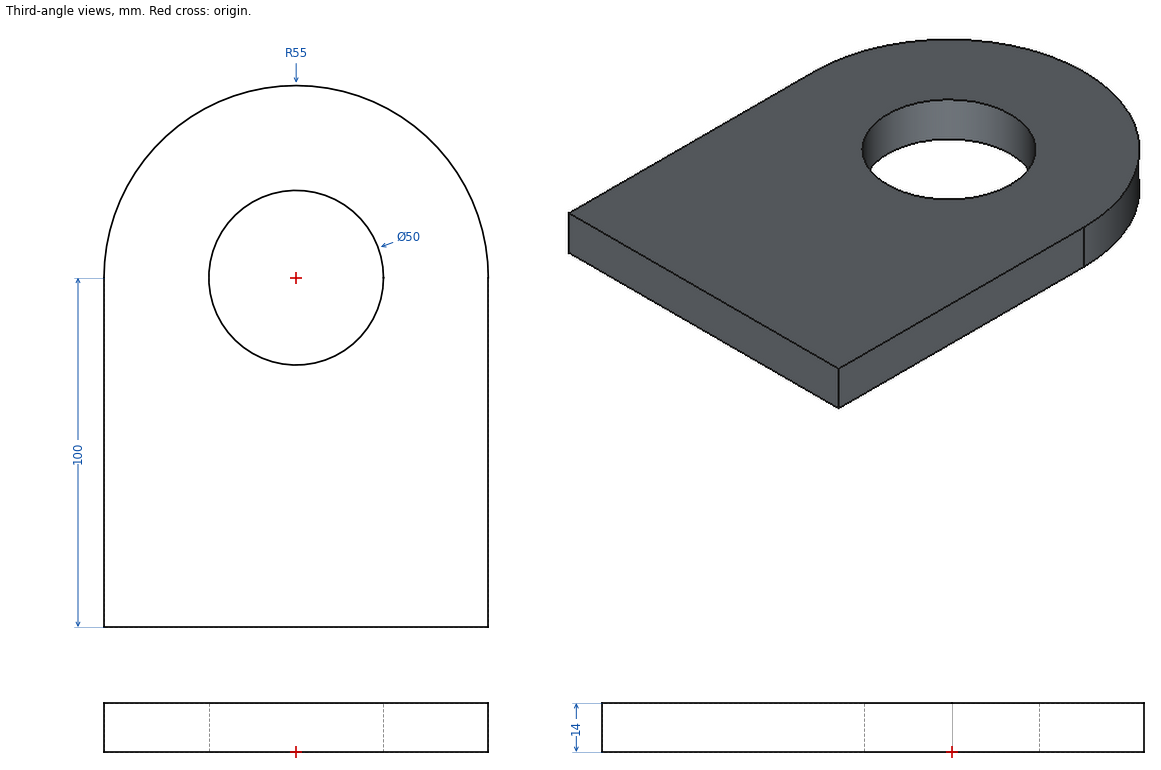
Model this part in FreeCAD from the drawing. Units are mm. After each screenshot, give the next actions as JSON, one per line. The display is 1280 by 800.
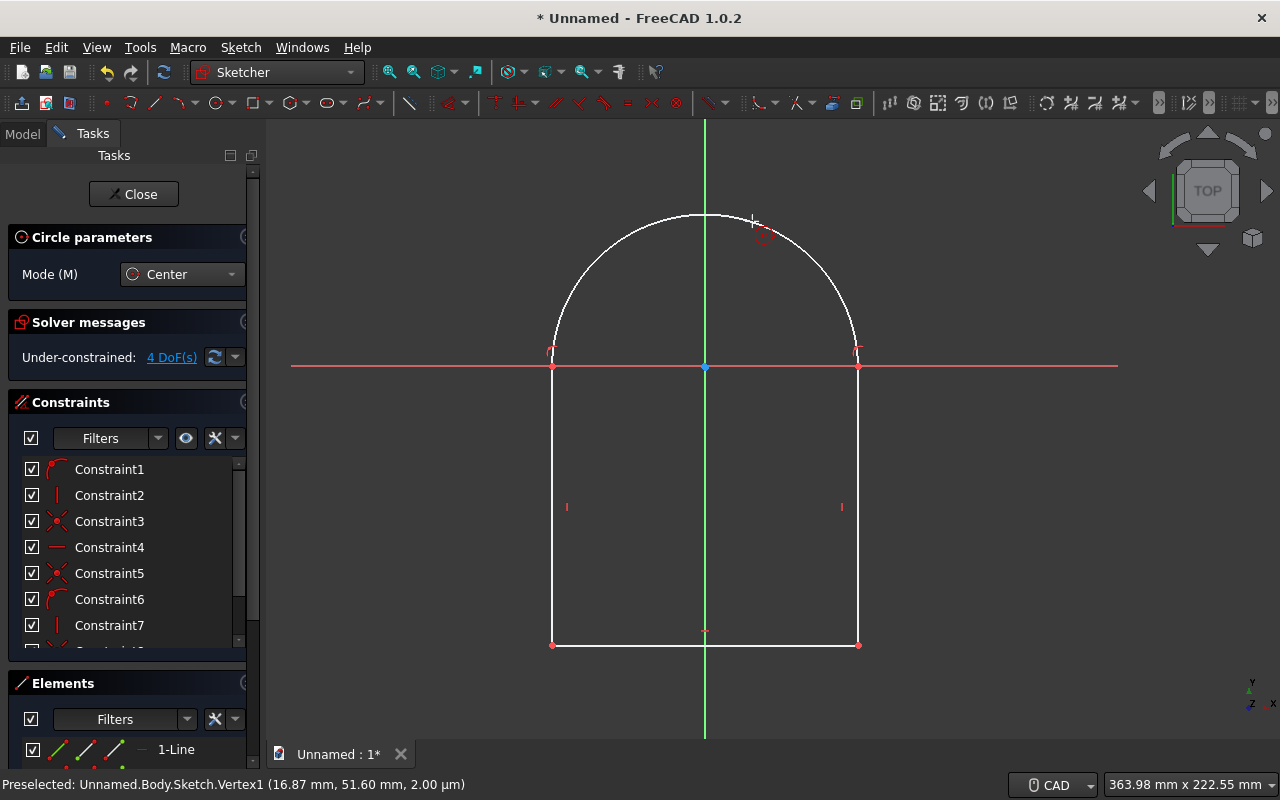
{"action": "left_click", "coordinate": [705, 366]}
{"action": "mouse_move", "coordinate": [754, 317]}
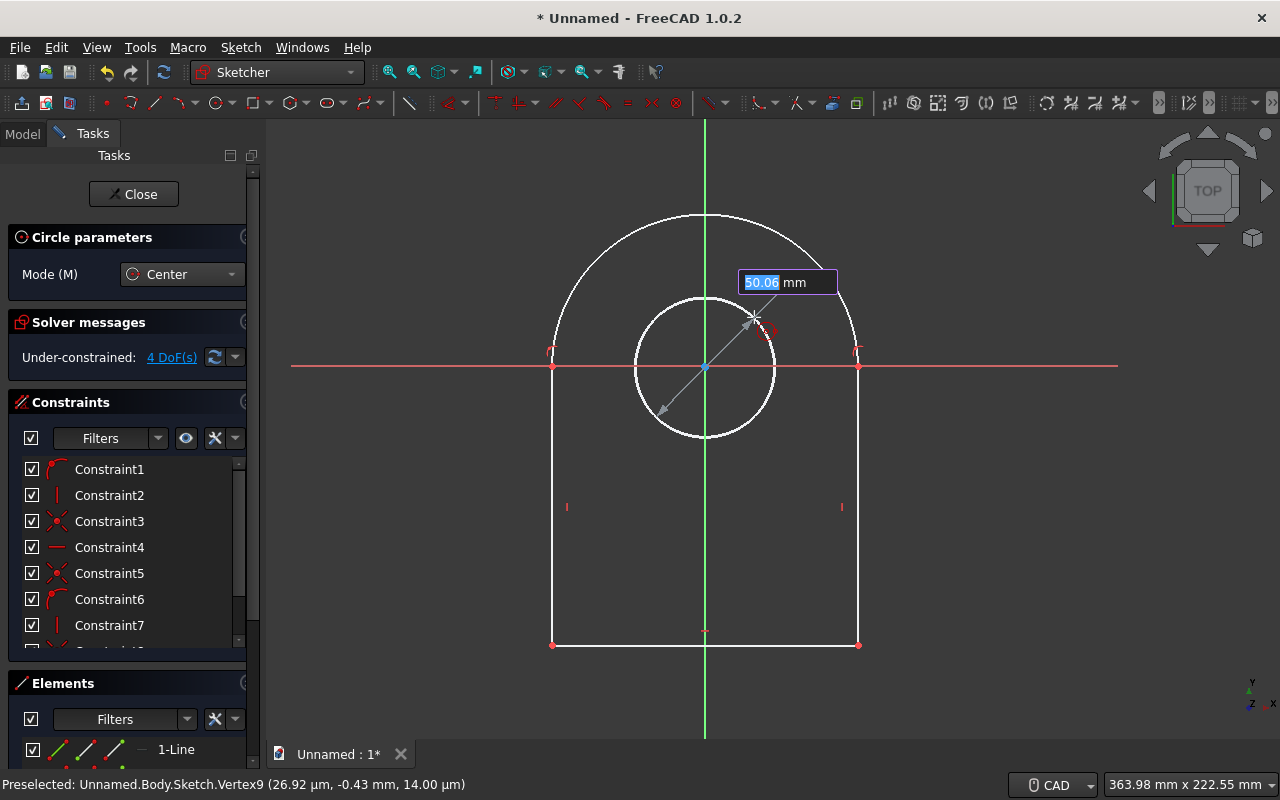
{"action": "type", "text": "50"}
{"action": "key", "text": "Return"}
{"action": "key", "text": "Escape"}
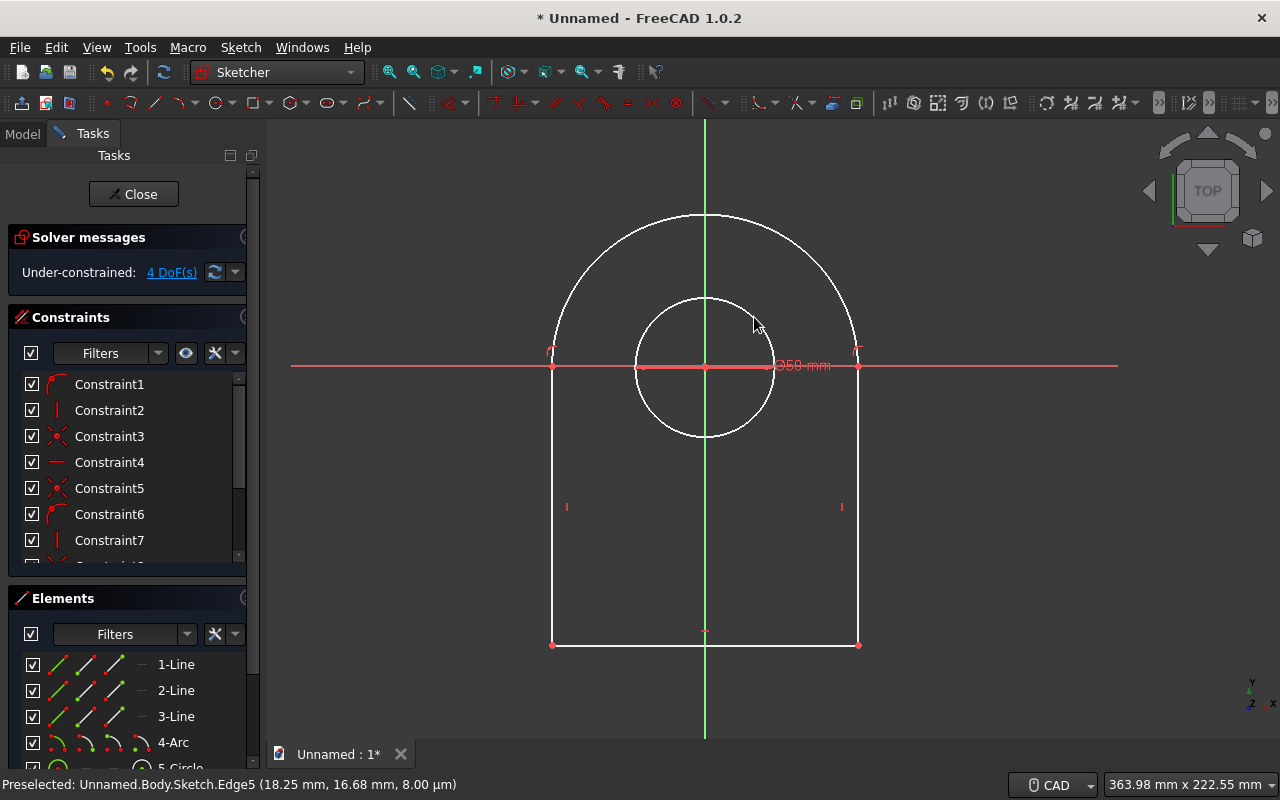
{"action": "left_click_drag", "start_coordinate": [695, 356], "coordinate": [715, 378]}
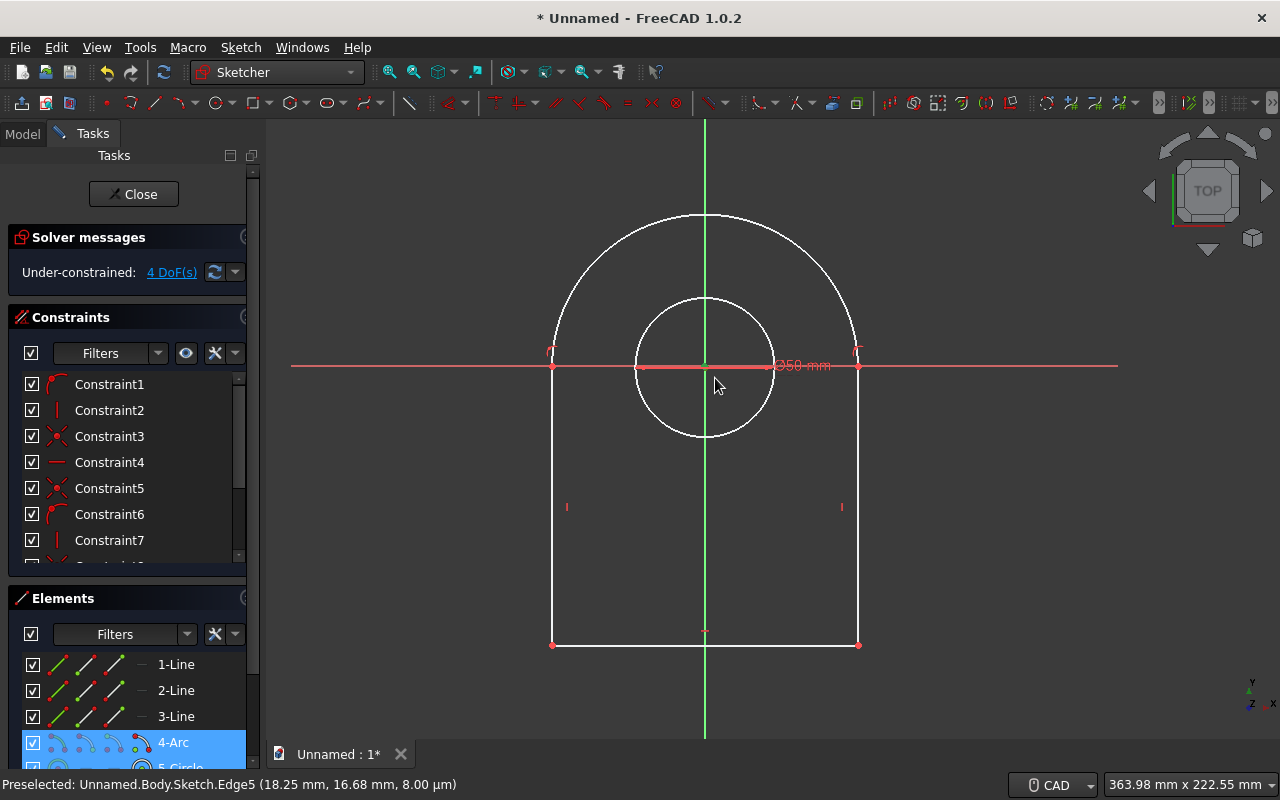
{"action": "key", "text": "c"}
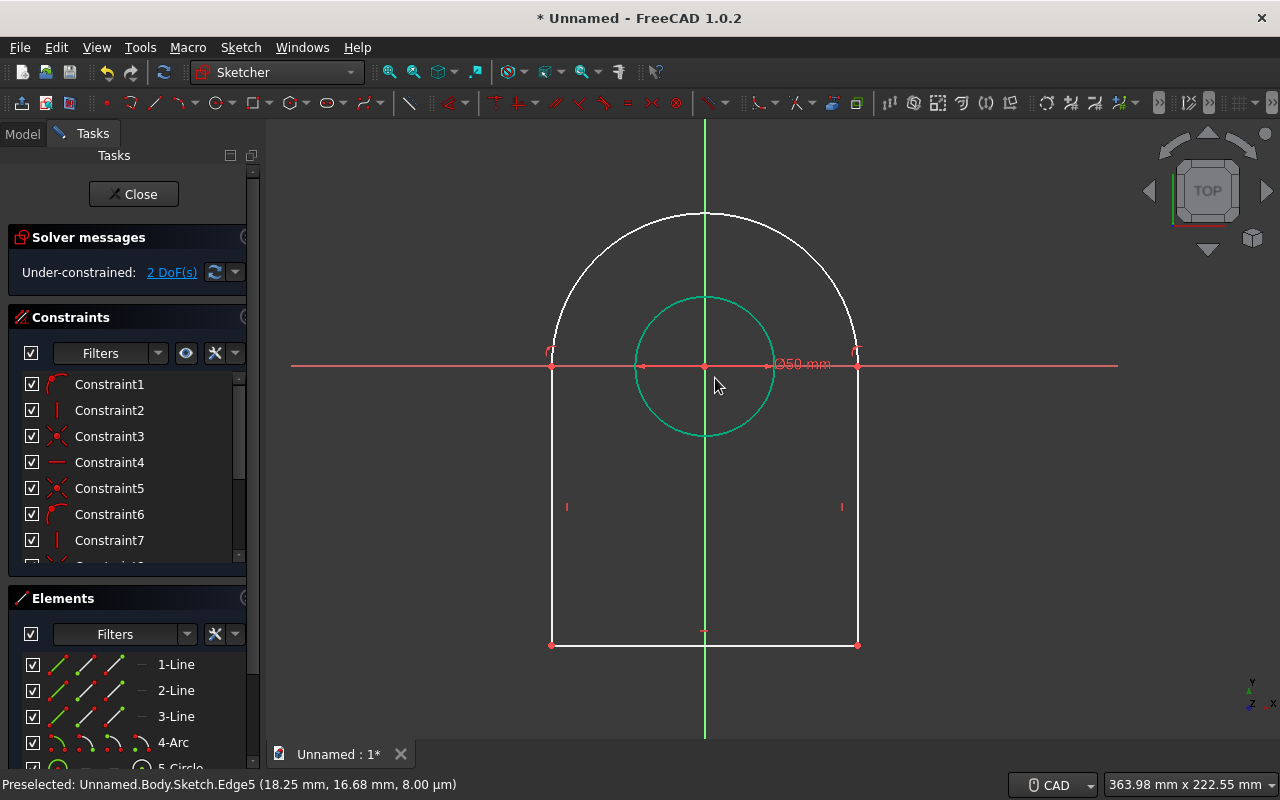
{"action": "left_click", "coordinate": [795, 243]}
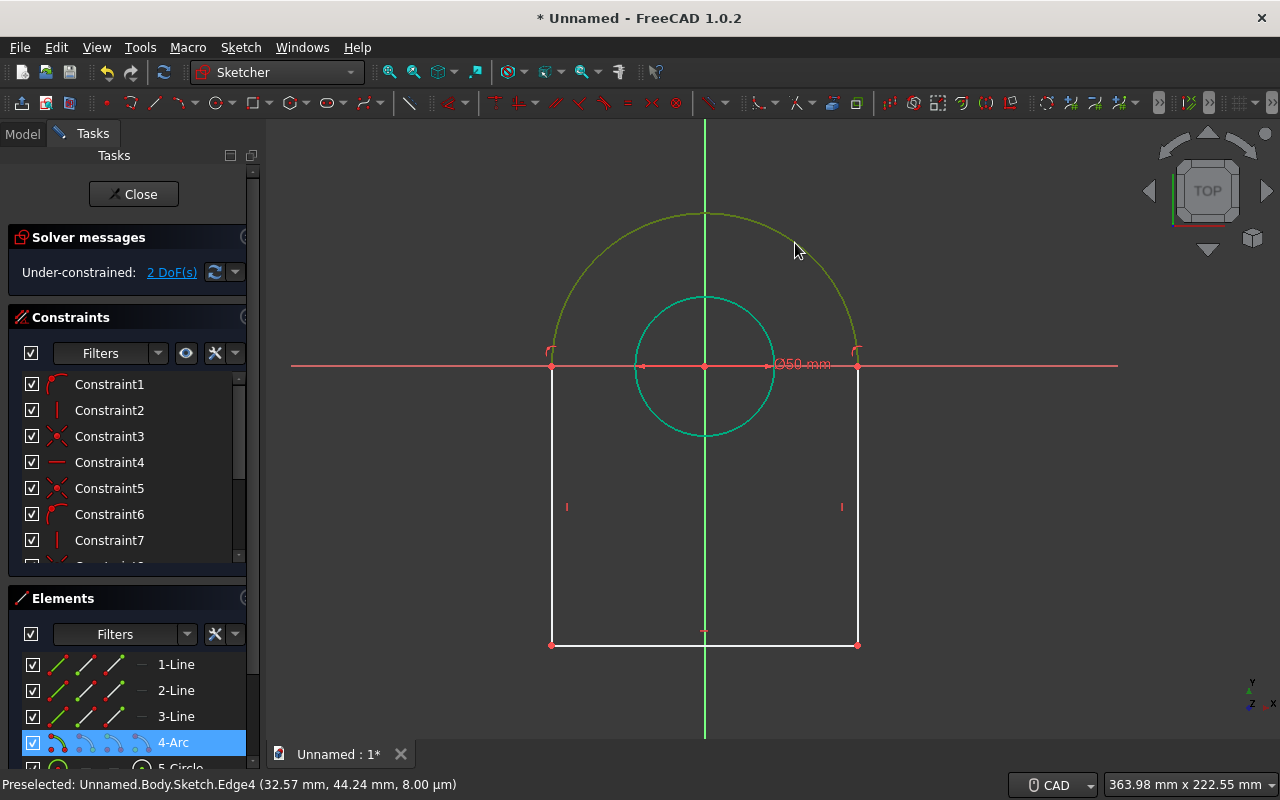
{"action": "left_click", "coordinate": [468, 104]}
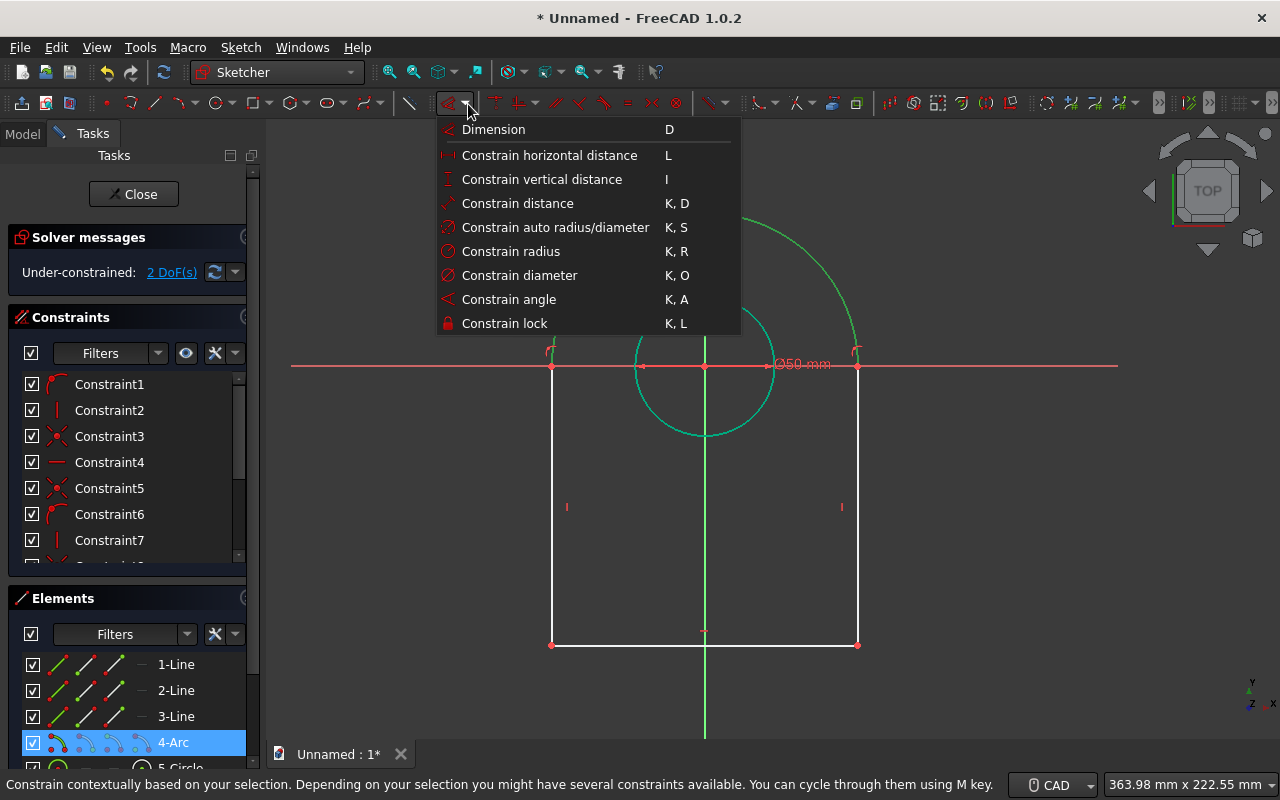
{"action": "left_click", "coordinate": [589, 251]}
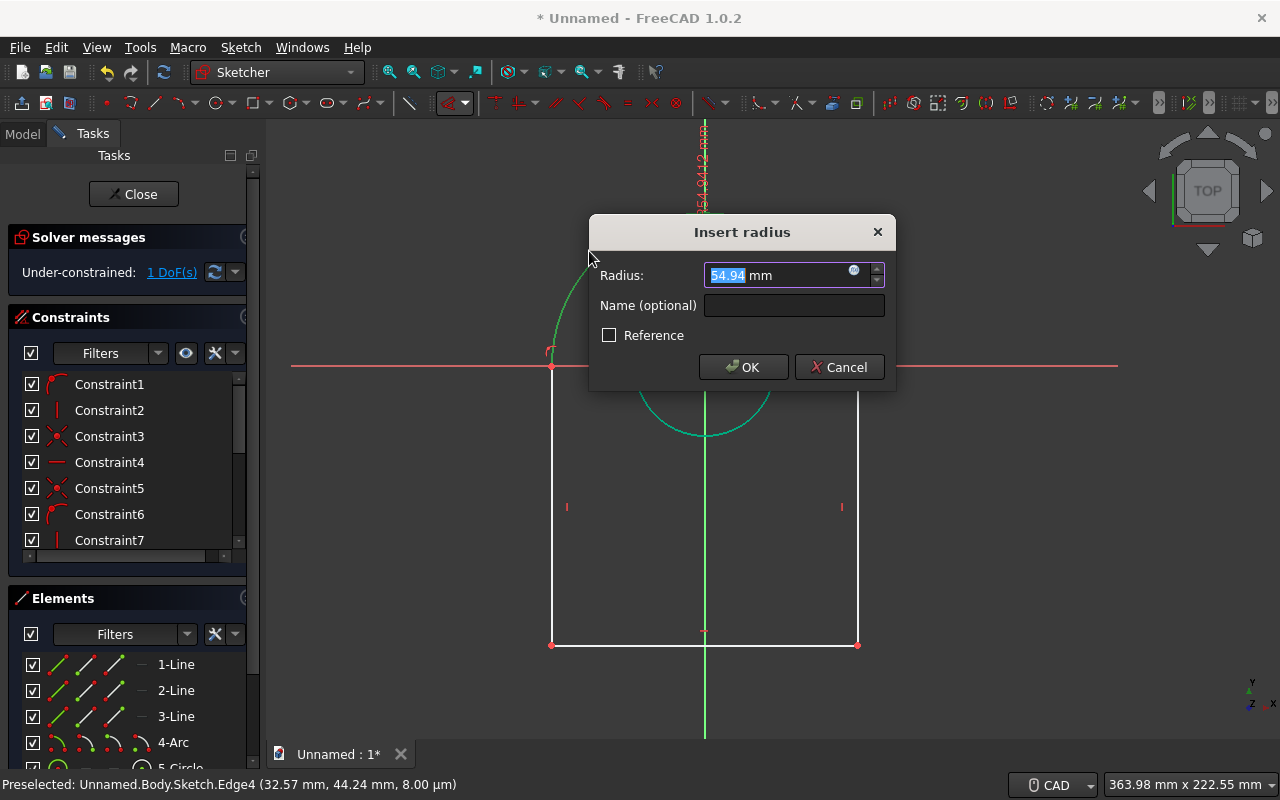
{"action": "type", "text": "55"}
{"action": "key", "text": "Return"}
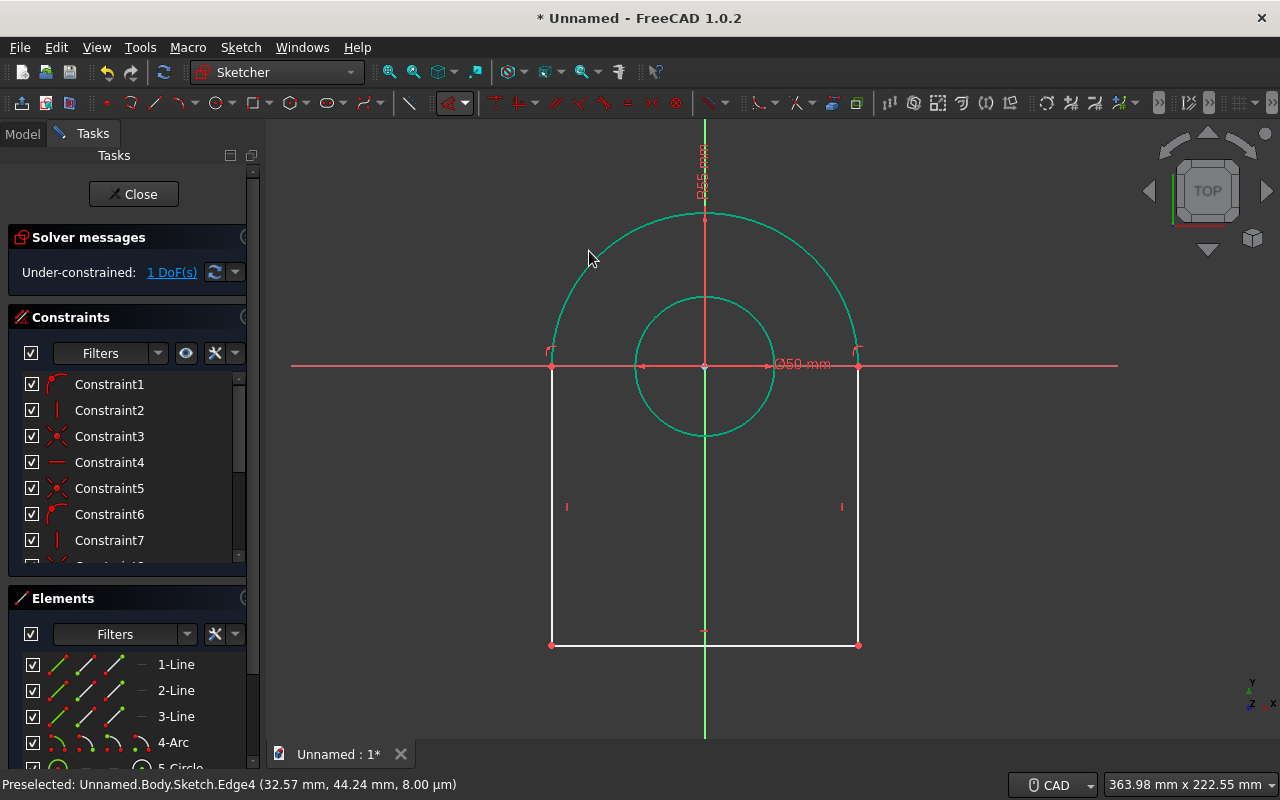
{"action": "left_click", "coordinate": [552, 450]}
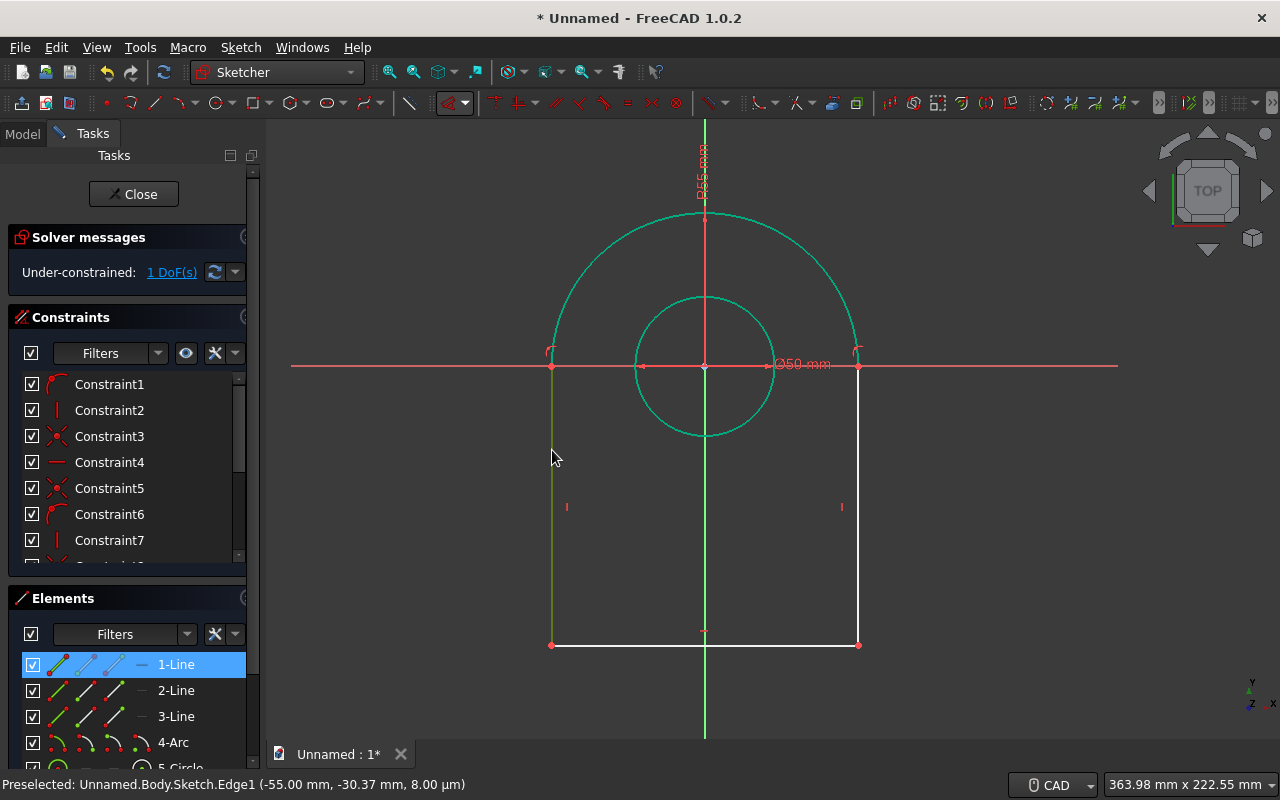
{"action": "key", "text": "i"}